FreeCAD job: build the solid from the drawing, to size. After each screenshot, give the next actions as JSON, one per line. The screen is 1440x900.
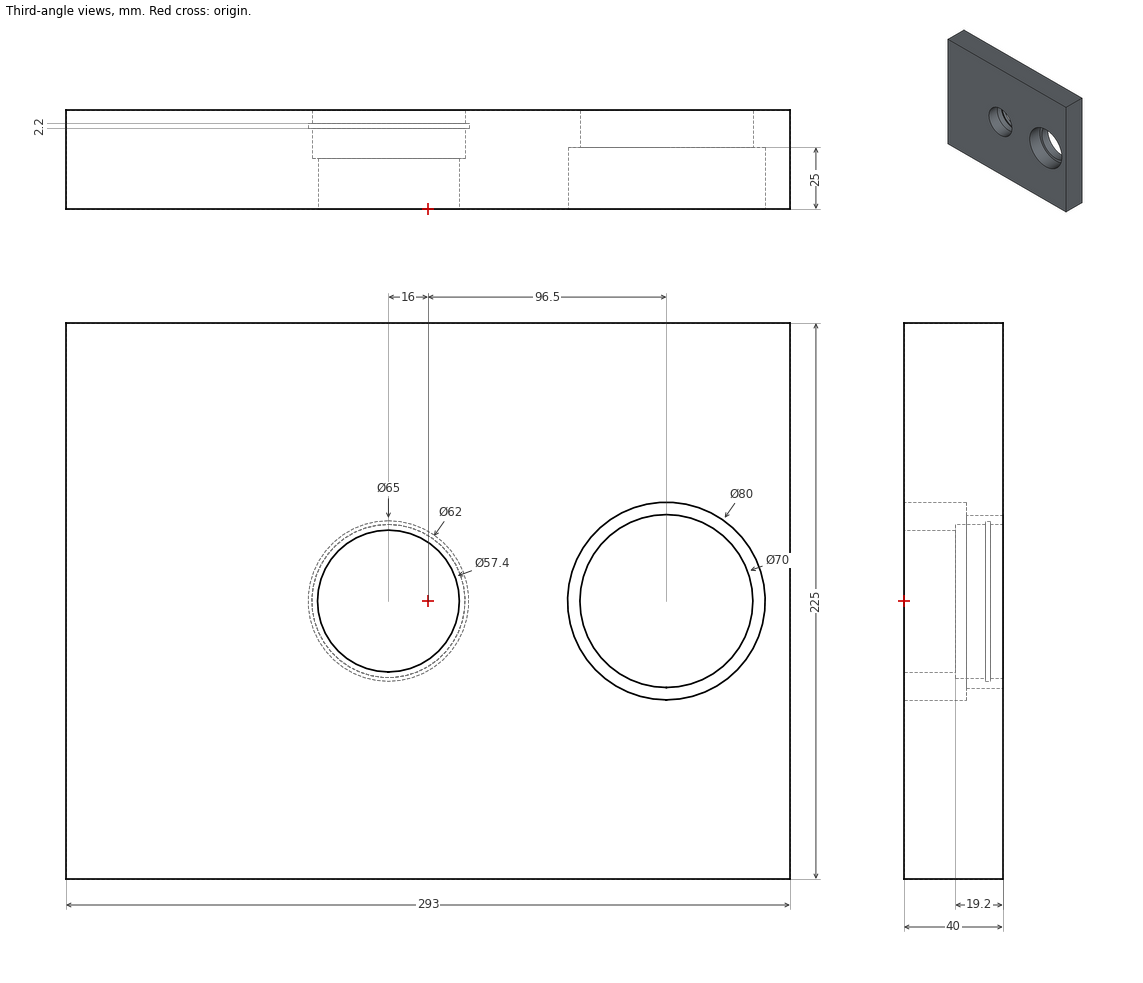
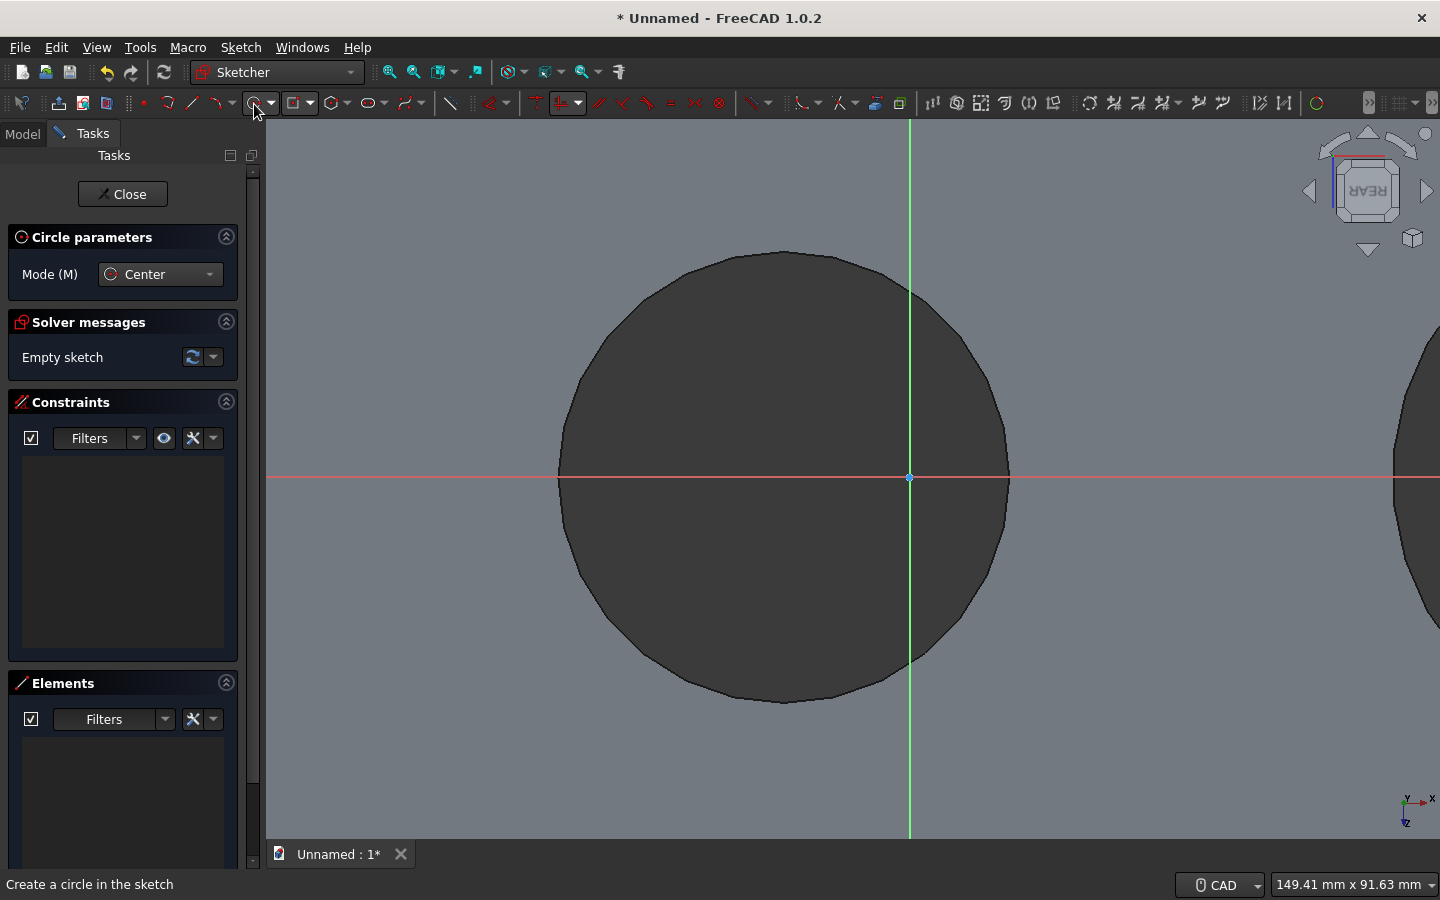
{"action": "left_click", "coordinate": [784, 477]}
{"action": "mouse_move", "coordinate": [956, 305]}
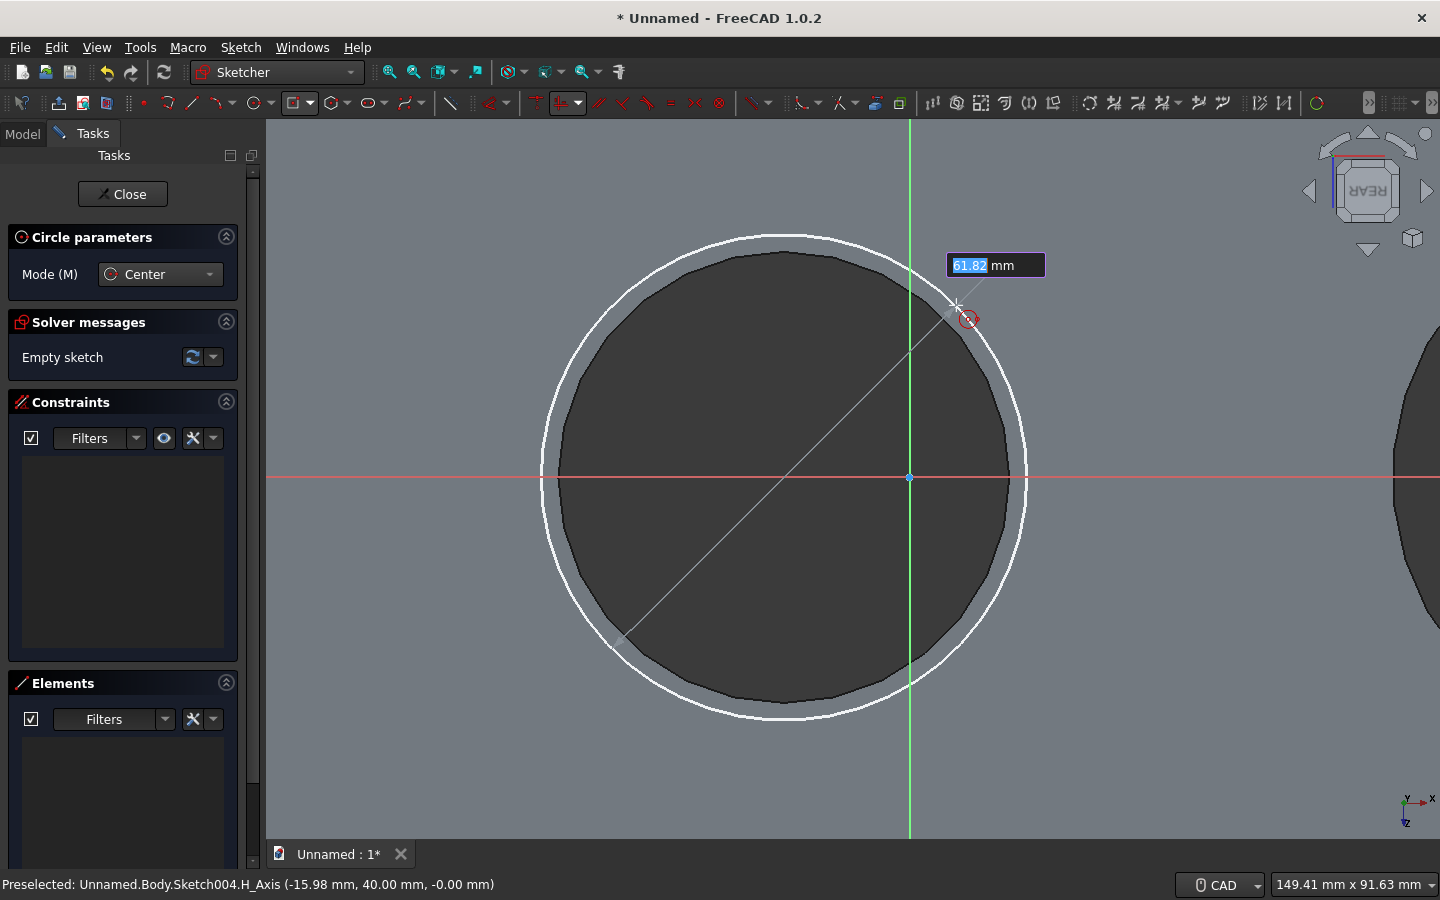
{"action": "type", "text": "62"}
{"action": "key", "text": "Return"}
{"action": "key", "text": "Escape"}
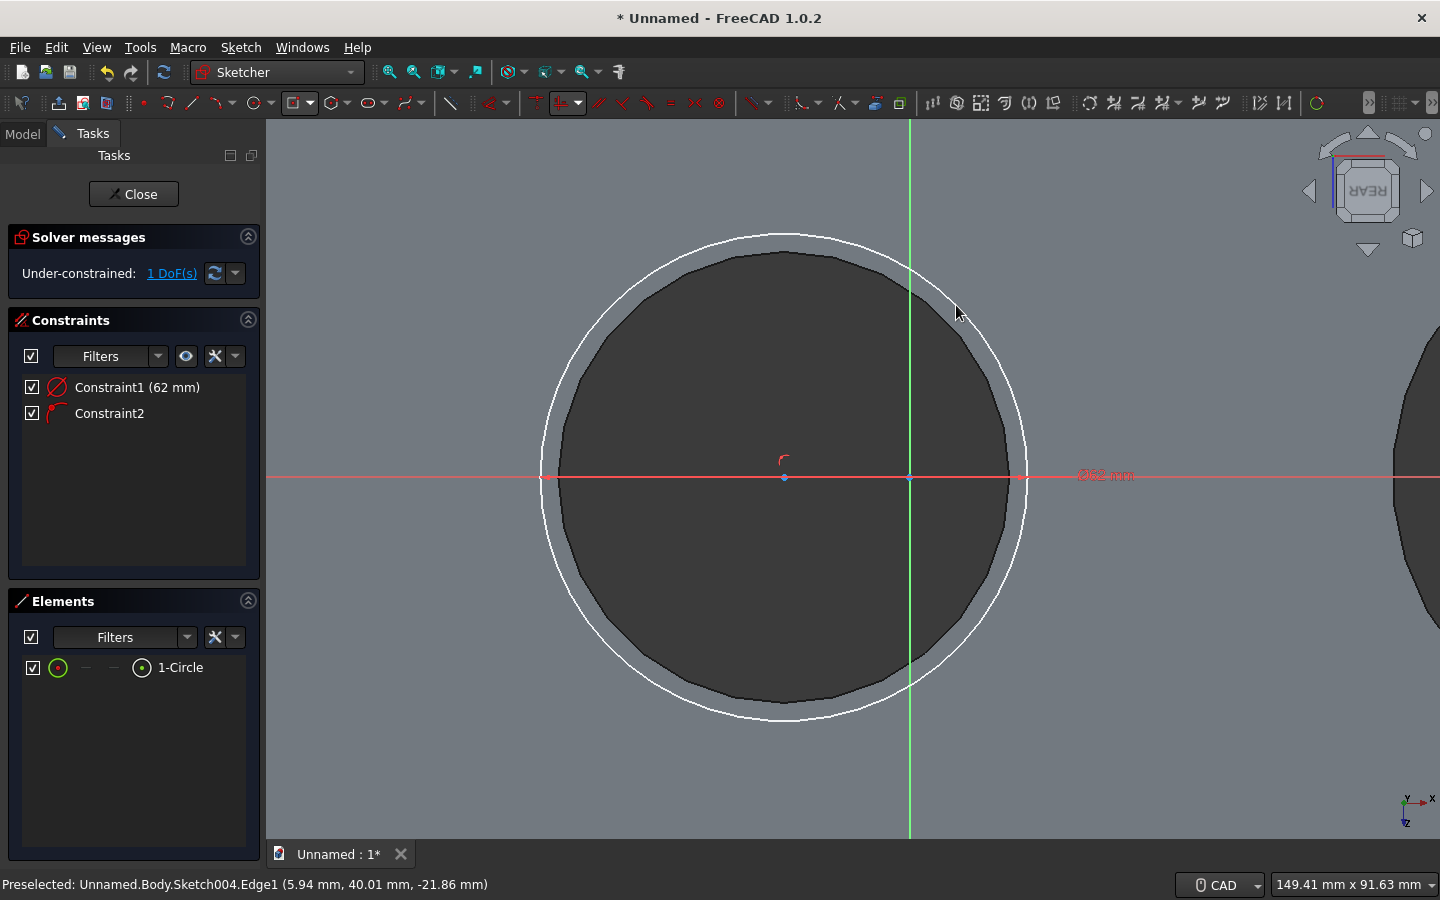
{"action": "left_click", "coordinate": [490, 104]}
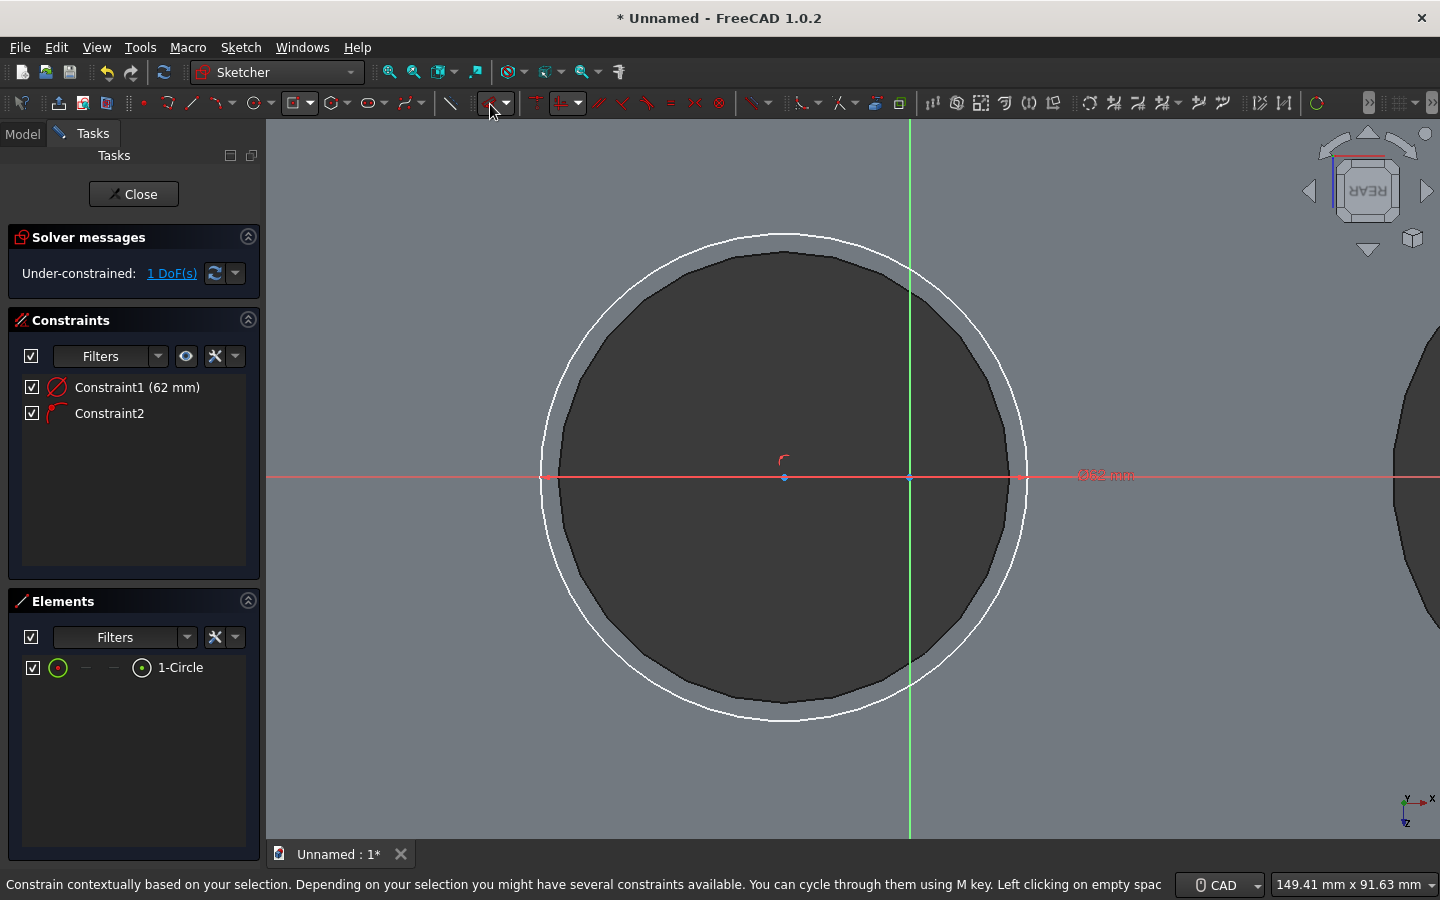
{"action": "left_click", "coordinate": [784, 477]}
{"action": "left_click", "coordinate": [847, 511]}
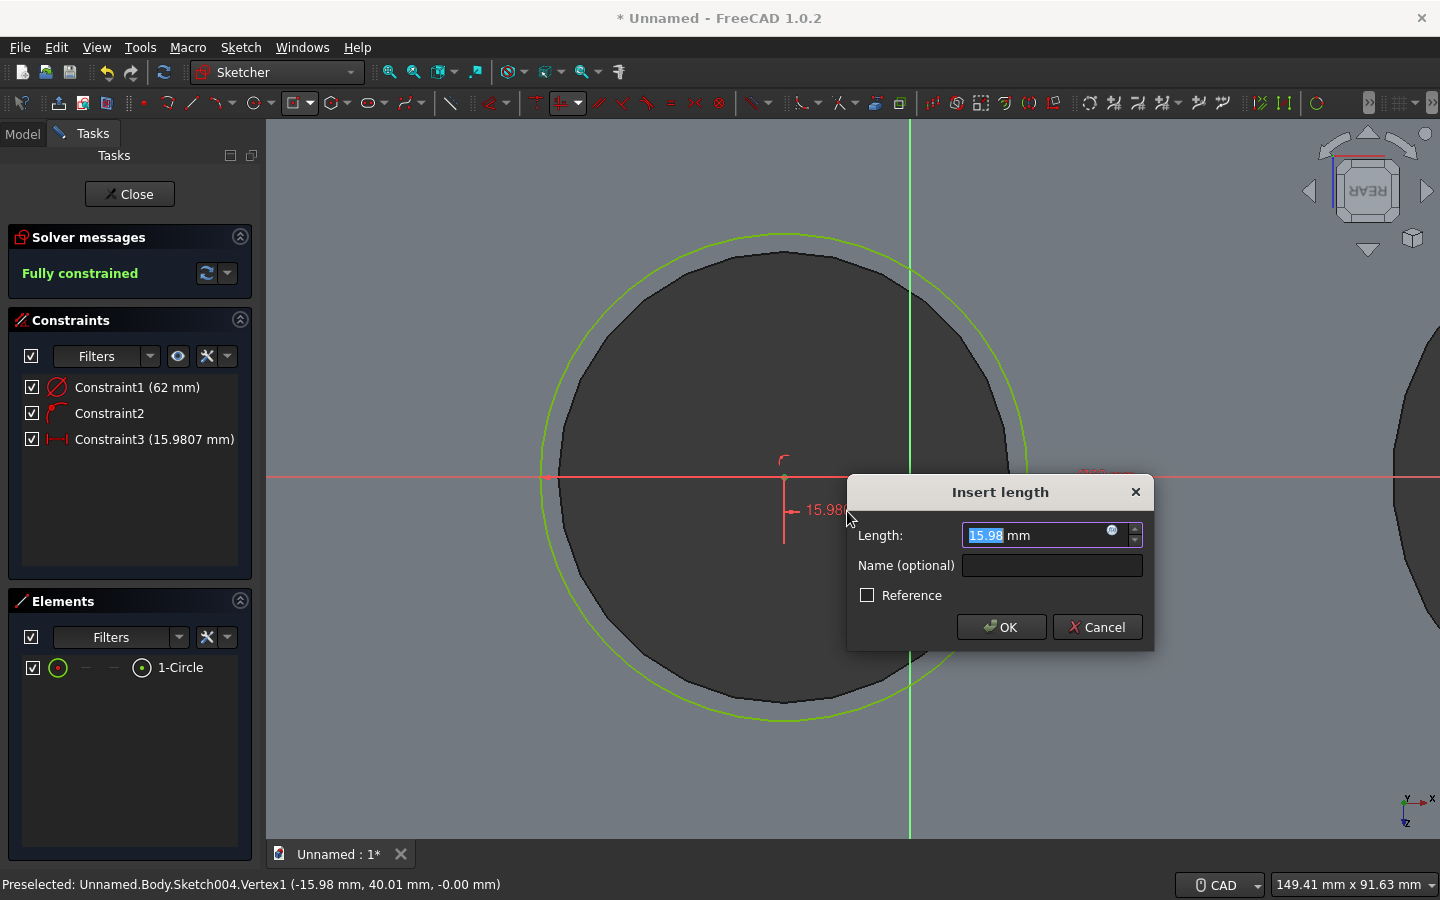
{"action": "type", "text": "16"}
{"action": "key", "text": "Return"}
{"action": "key", "text": "Escape"}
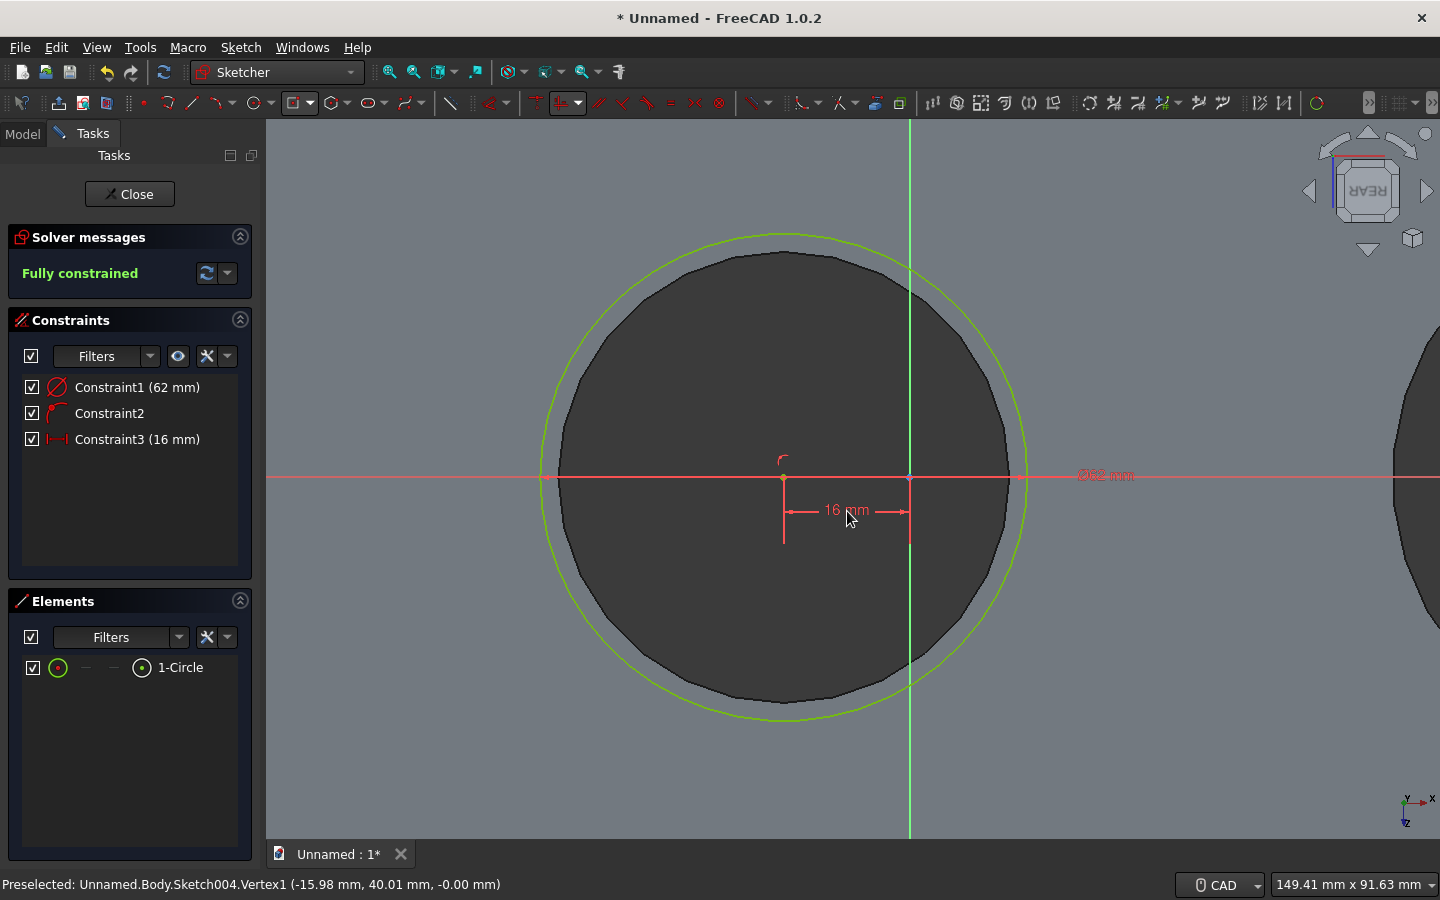
{"action": "left_click", "coordinate": [130, 194]}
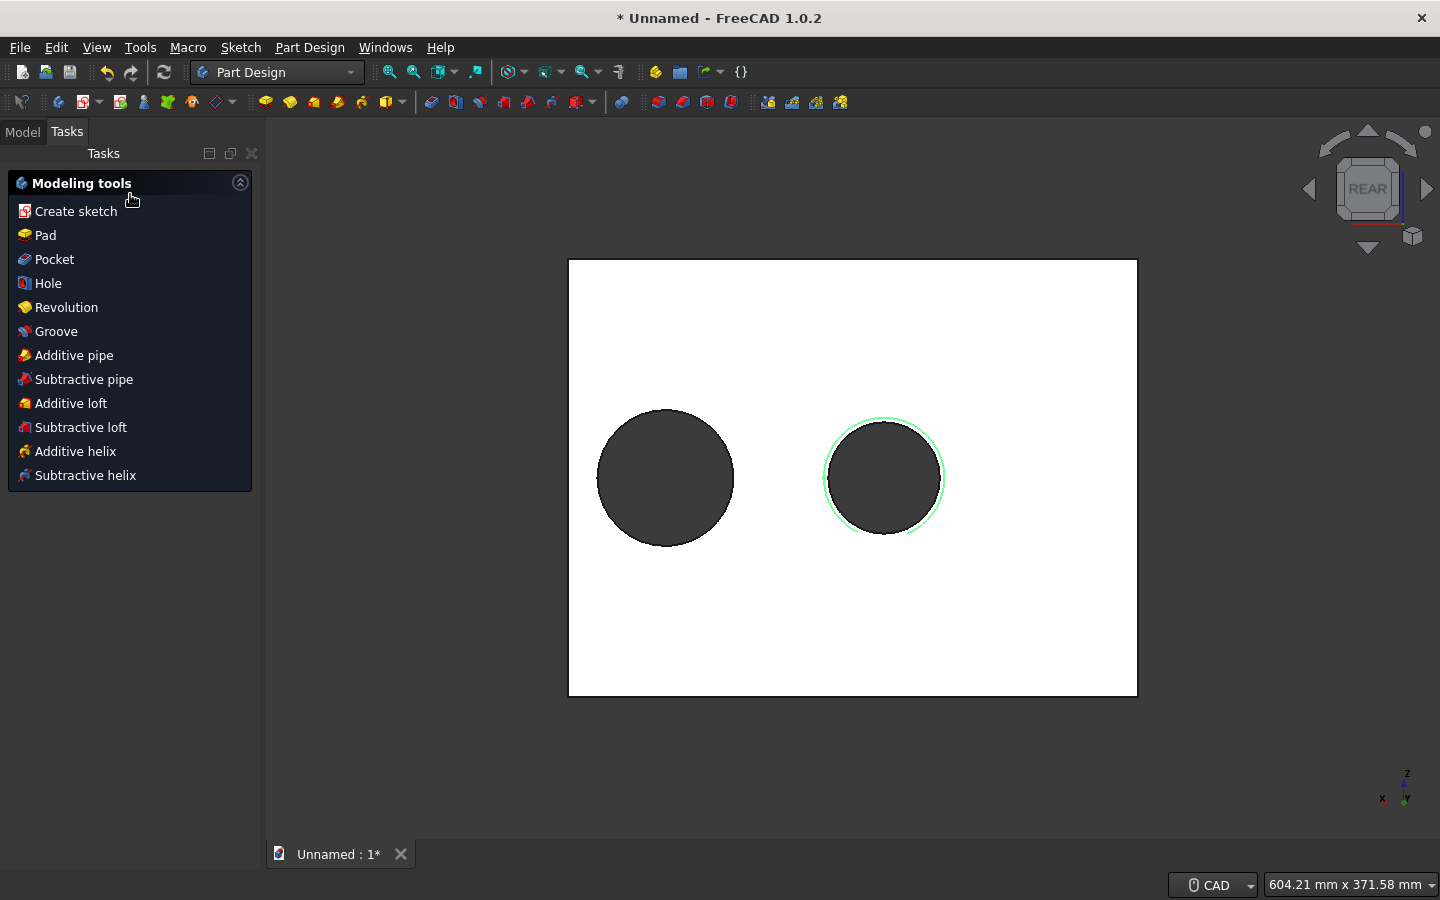
{"action": "left_click", "coordinate": [432, 102]}